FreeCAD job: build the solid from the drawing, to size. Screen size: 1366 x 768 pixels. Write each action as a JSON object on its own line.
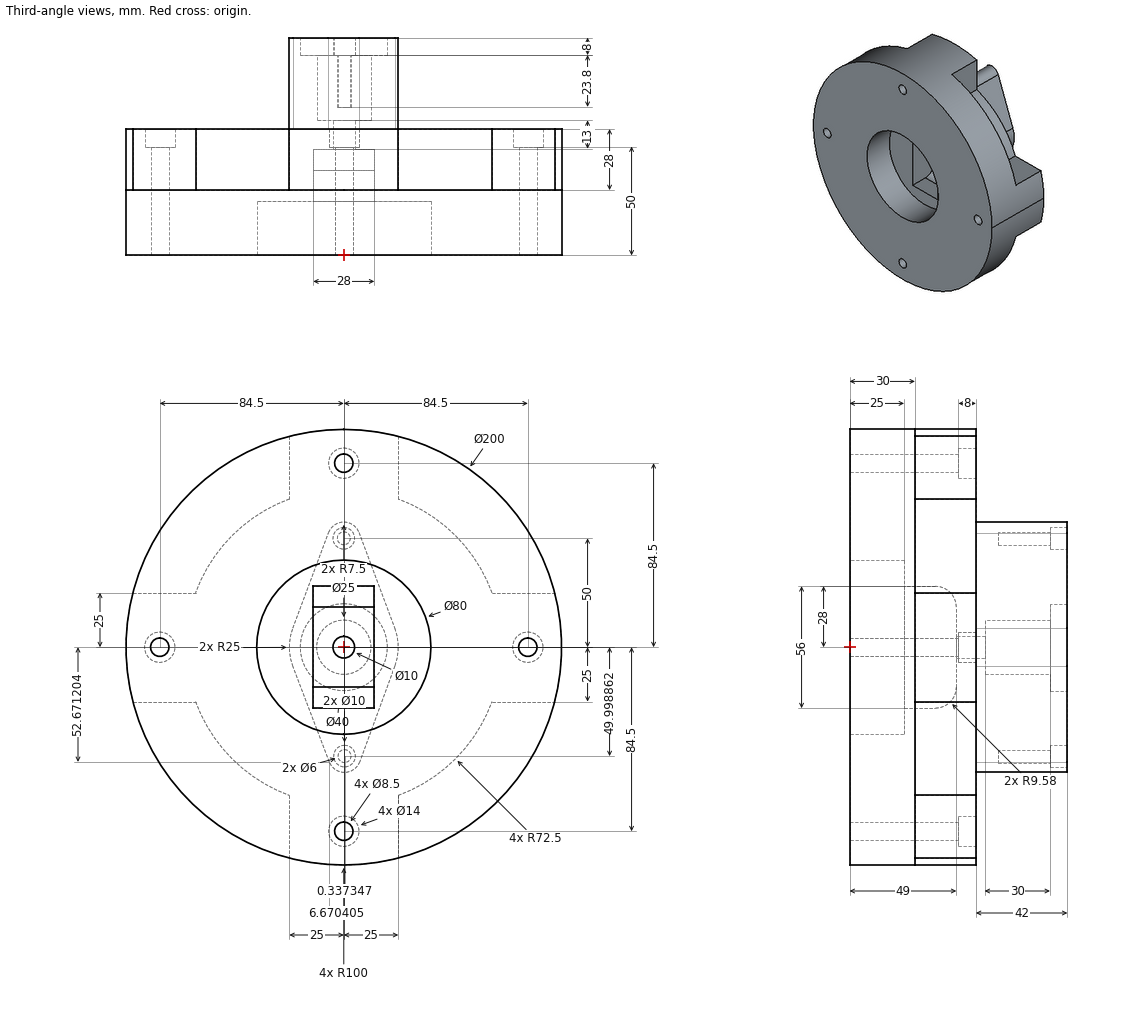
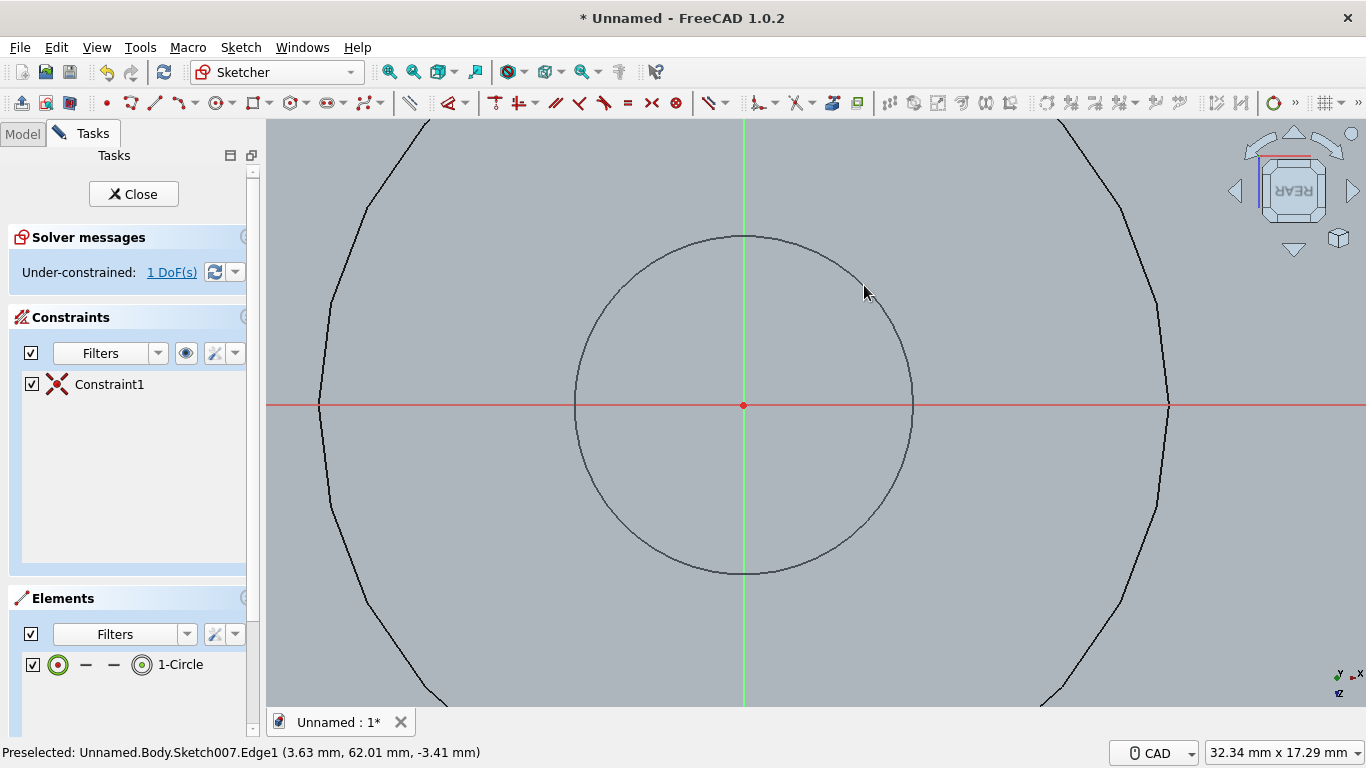
{"action": "key", "text": "d"}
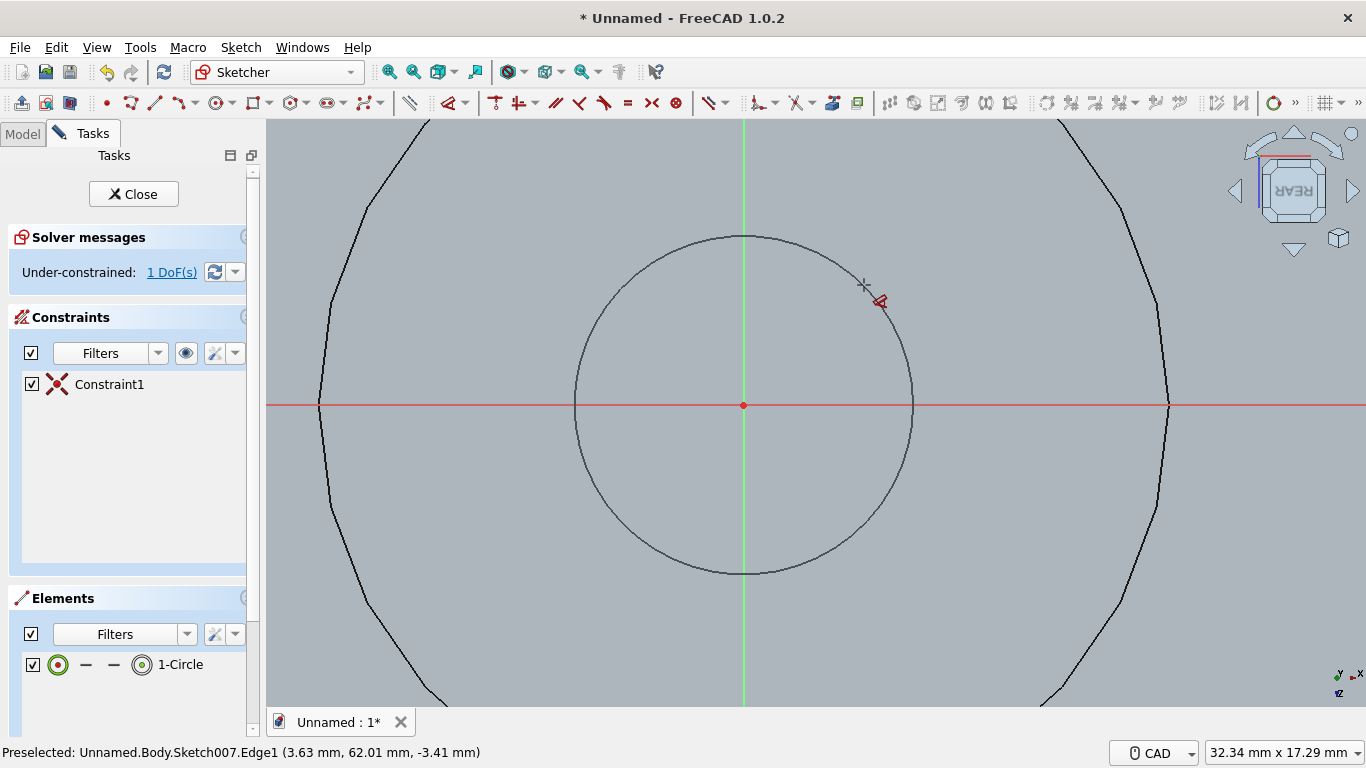
{"action": "left_click", "coordinate": [863, 285]}
{"action": "left_click", "coordinate": [886, 262]}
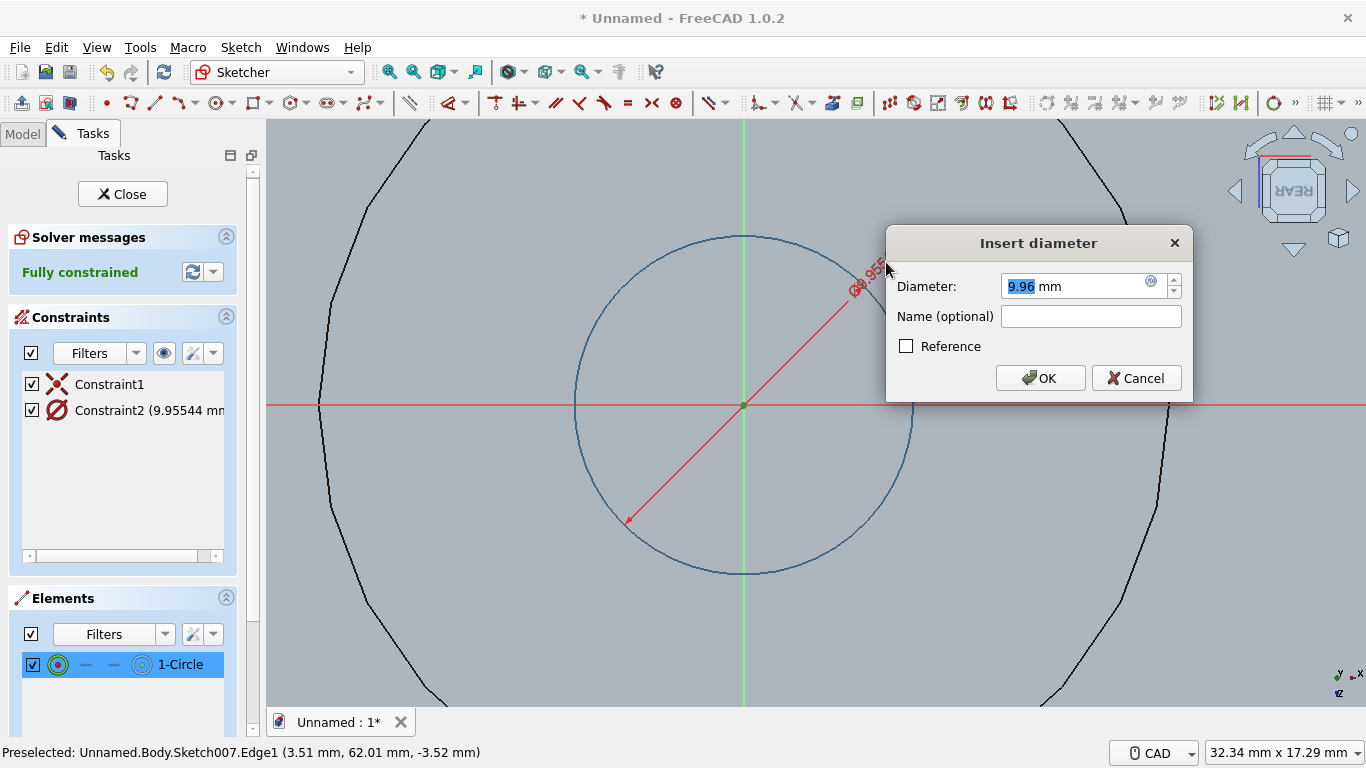
{"action": "type", "text": "10"}
{"action": "key", "text": "Return"}
{"action": "key", "text": "Escape"}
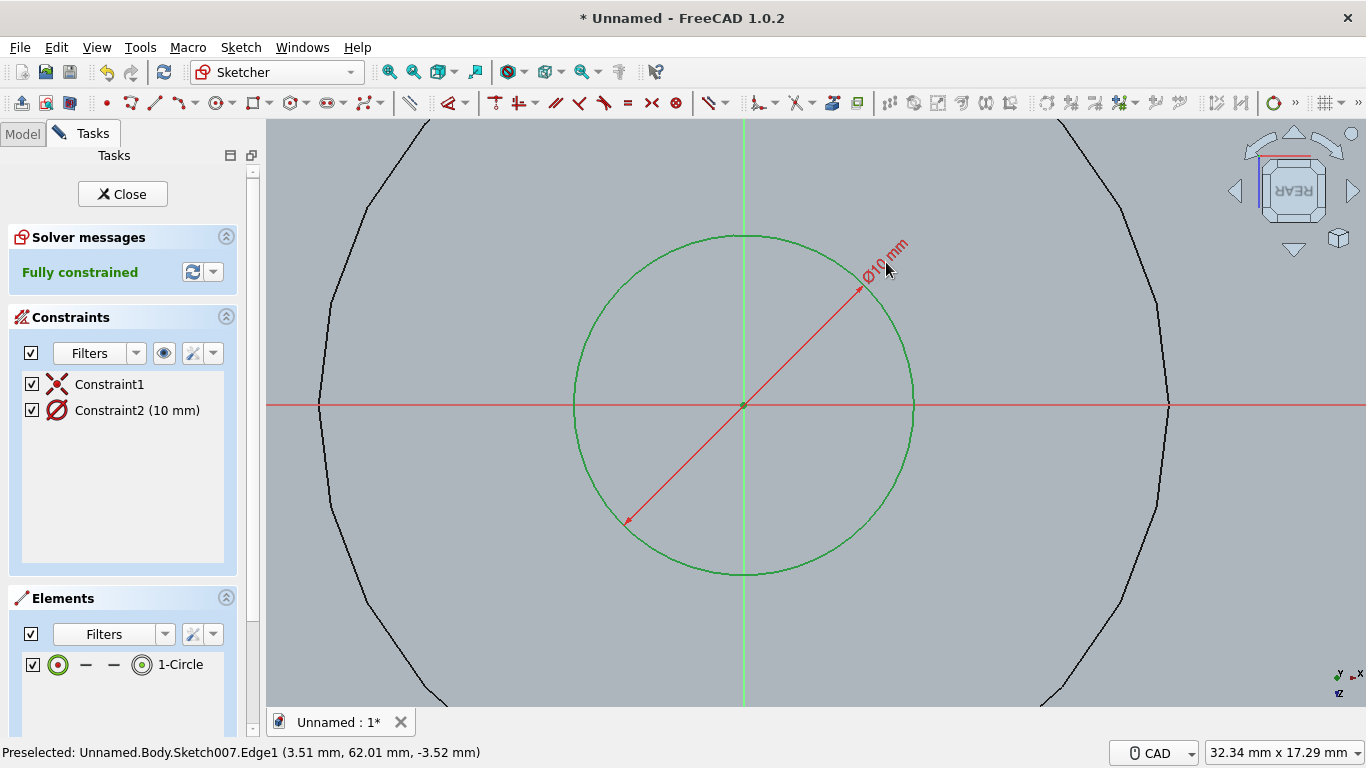
{"action": "left_click", "coordinate": [123, 194]}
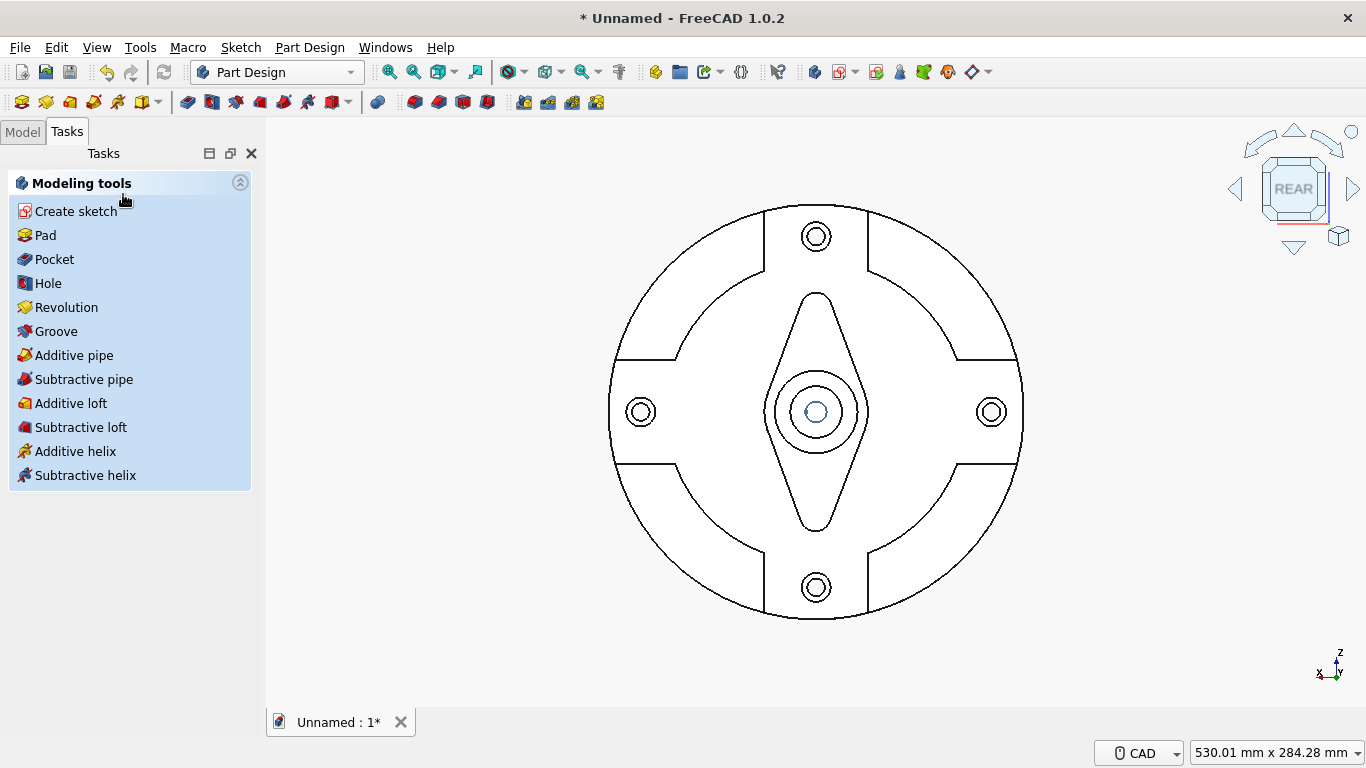
{"action": "left_click", "coordinate": [188, 102]}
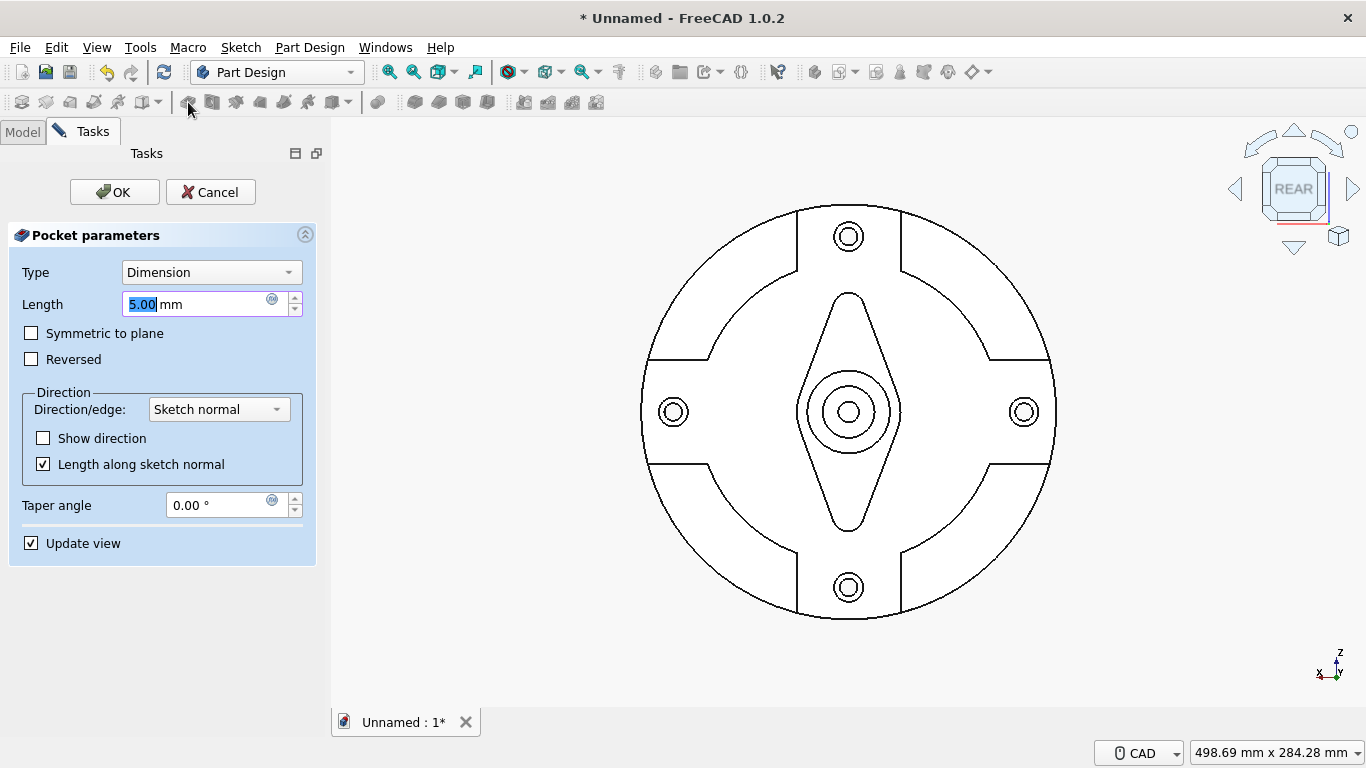
{"action": "type", "text": "13"}
{"action": "key", "text": "Tab"}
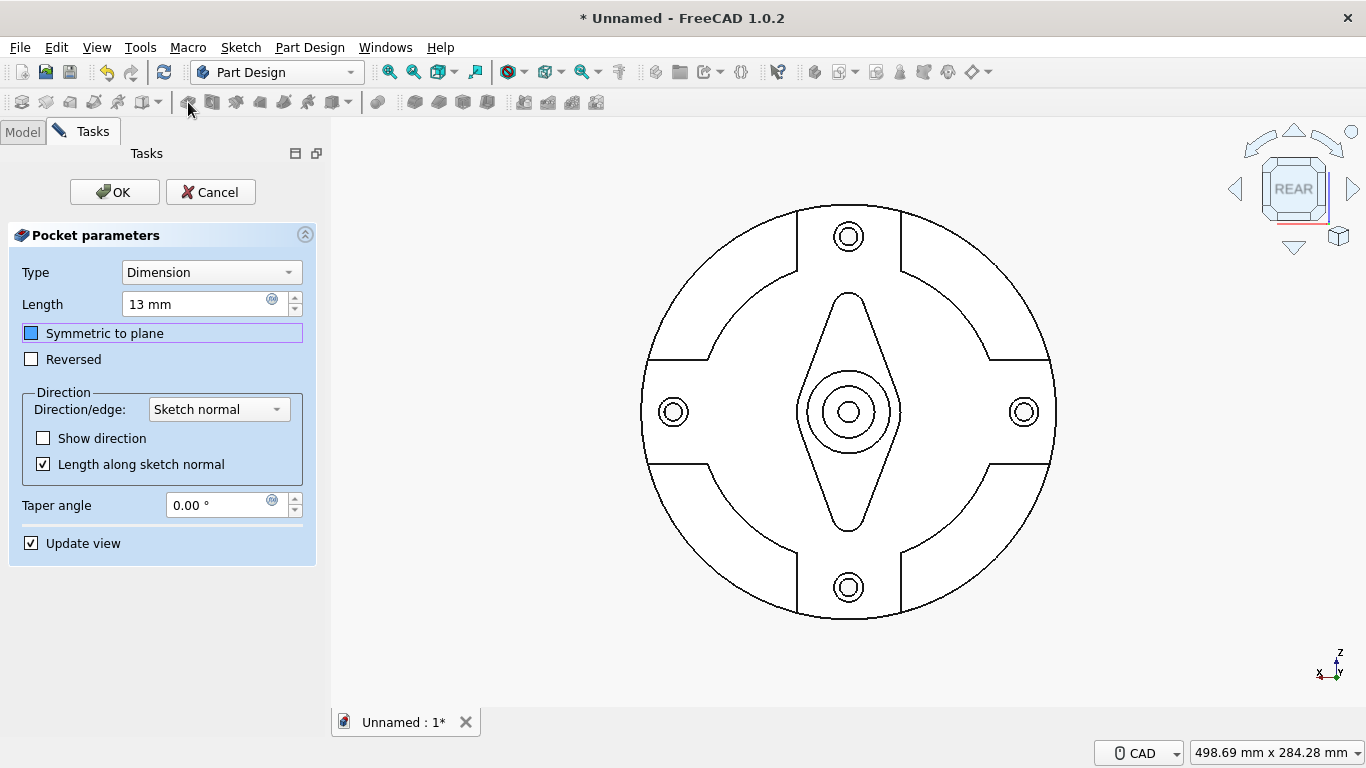
{"action": "left_click", "coordinate": [115, 192]}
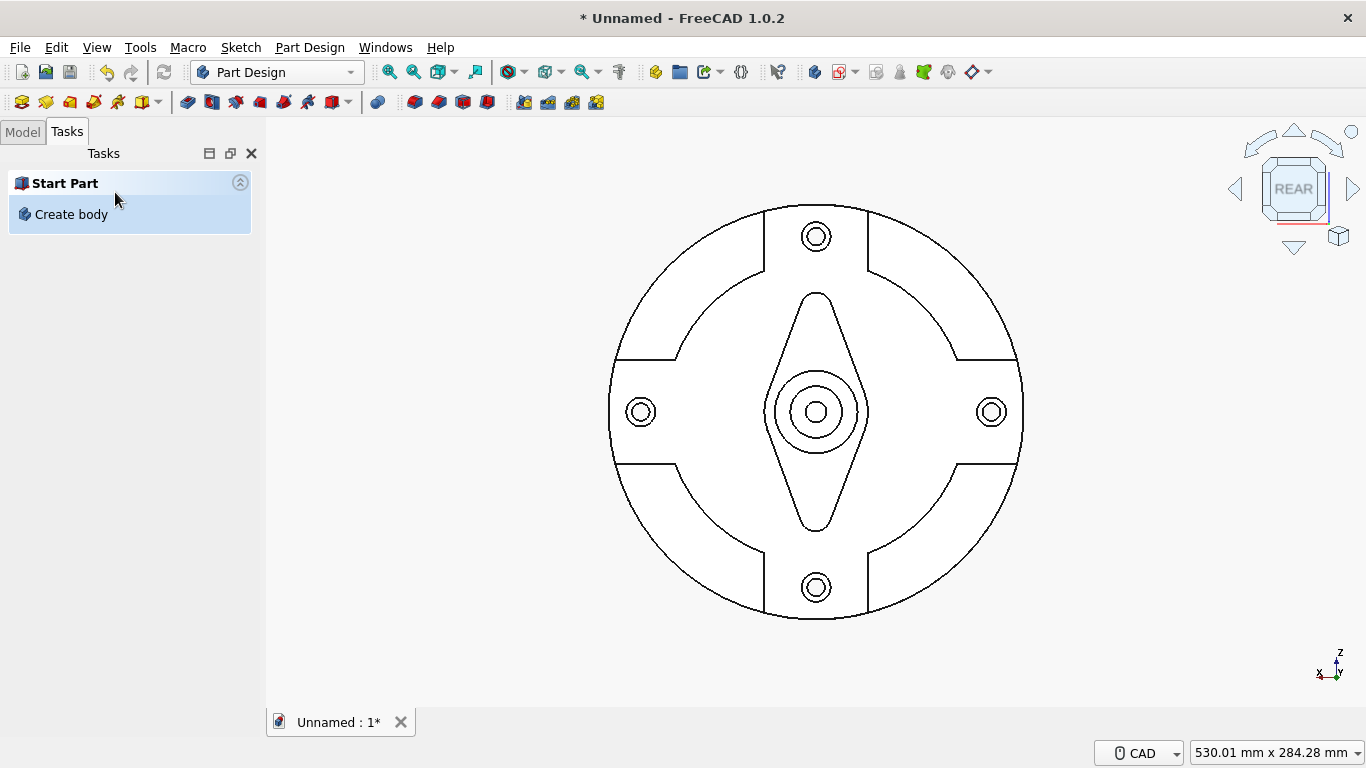
{"action": "key", "text": "0"}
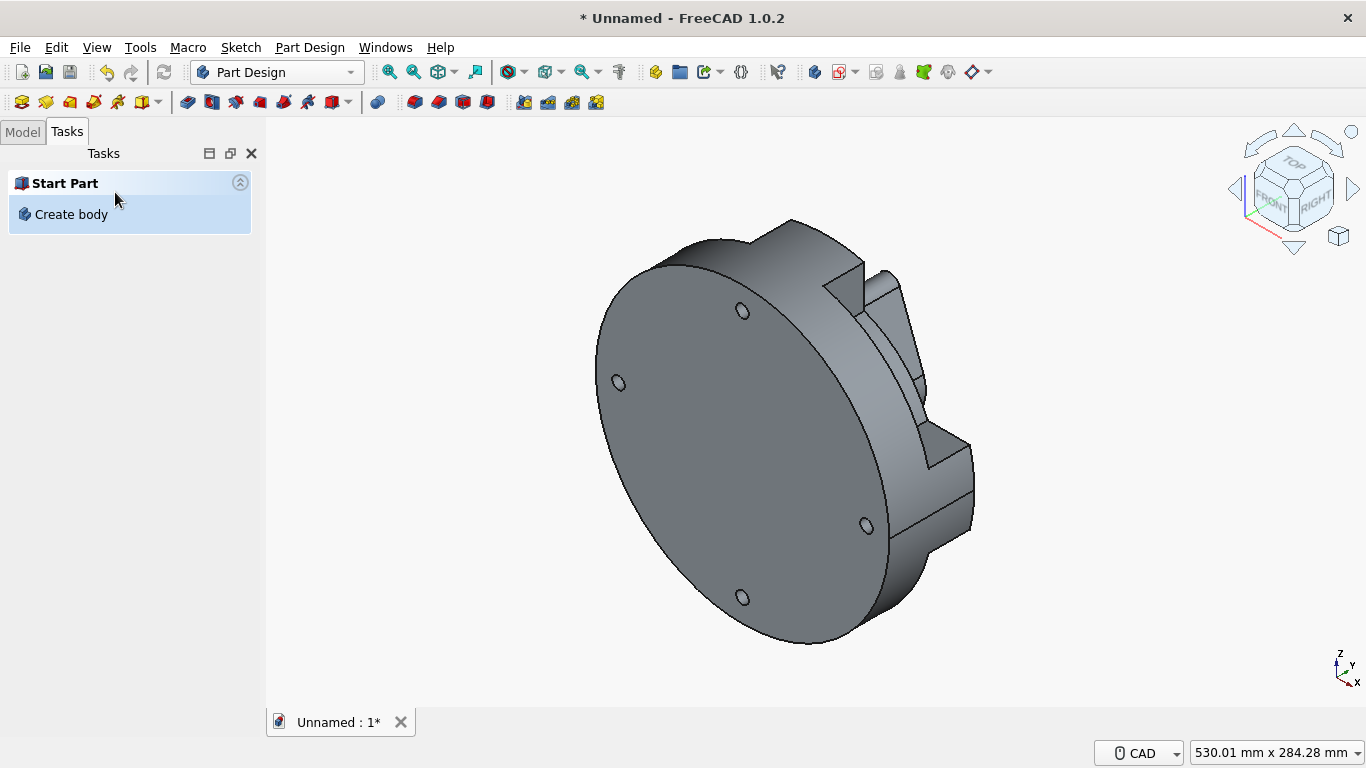
{"action": "key", "text": "v f"}